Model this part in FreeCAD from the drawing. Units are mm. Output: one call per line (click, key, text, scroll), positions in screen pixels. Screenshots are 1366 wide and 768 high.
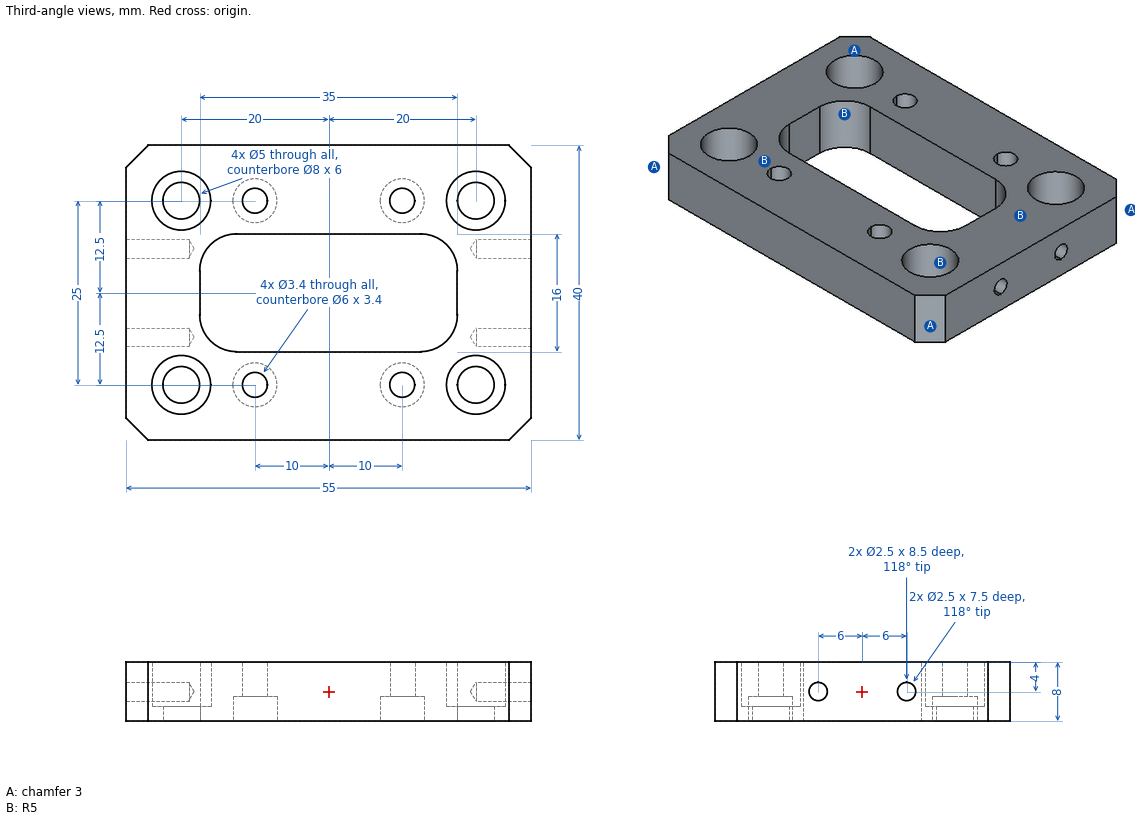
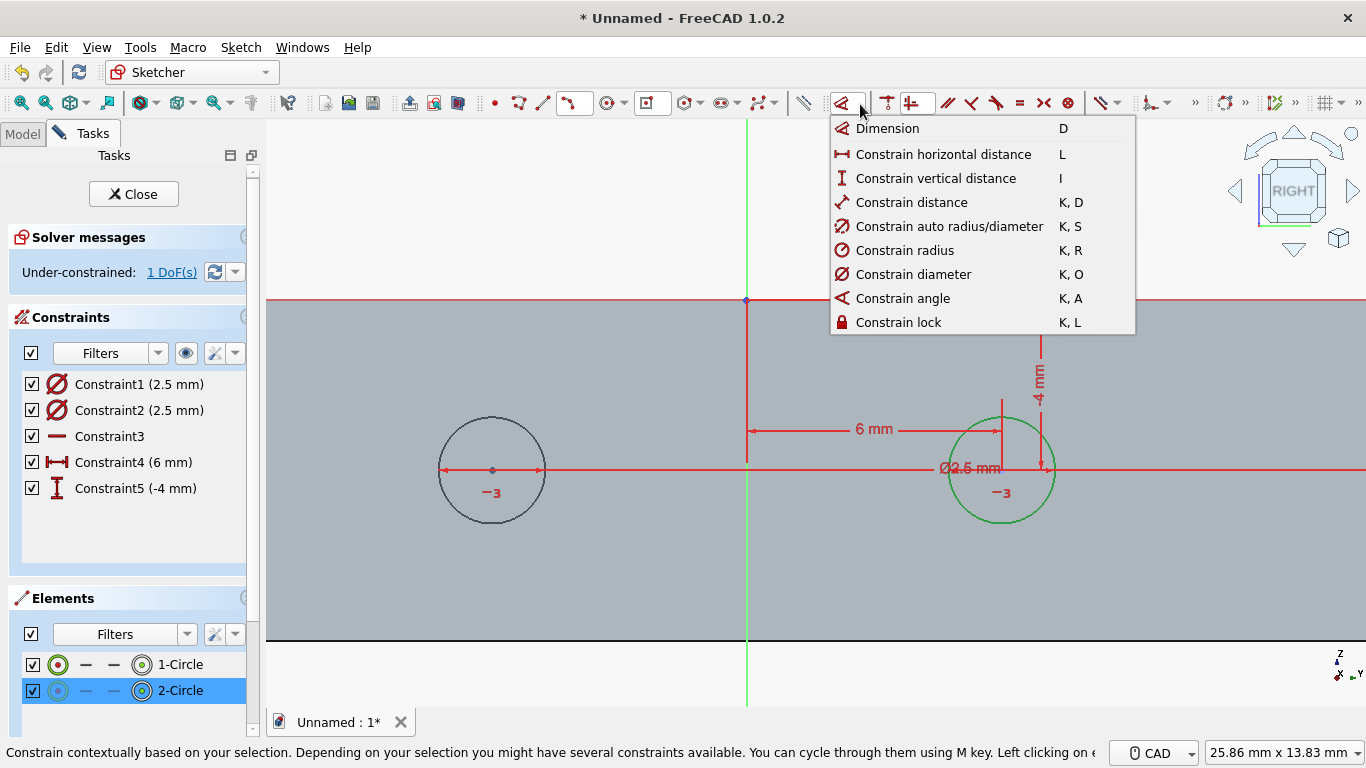
click(983, 154)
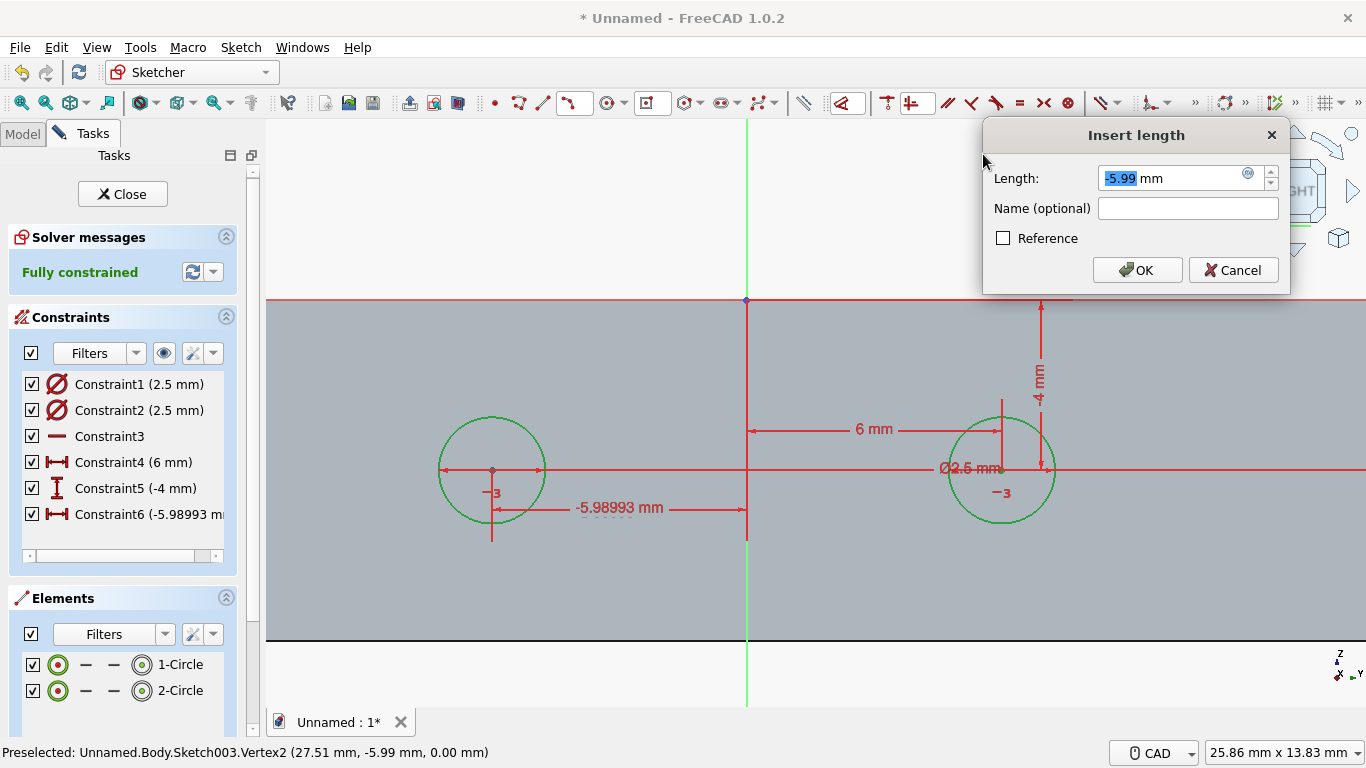
text(-6)
key(Return)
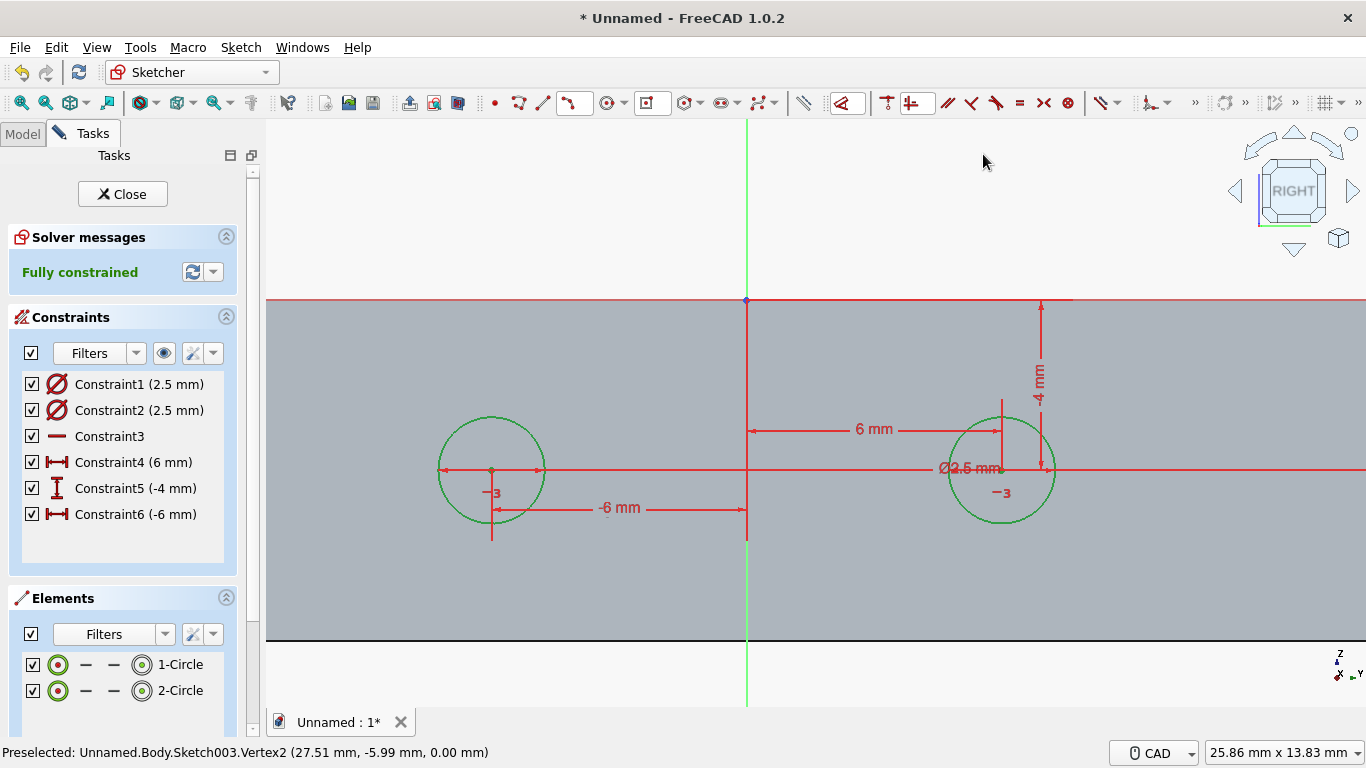
click(123, 194)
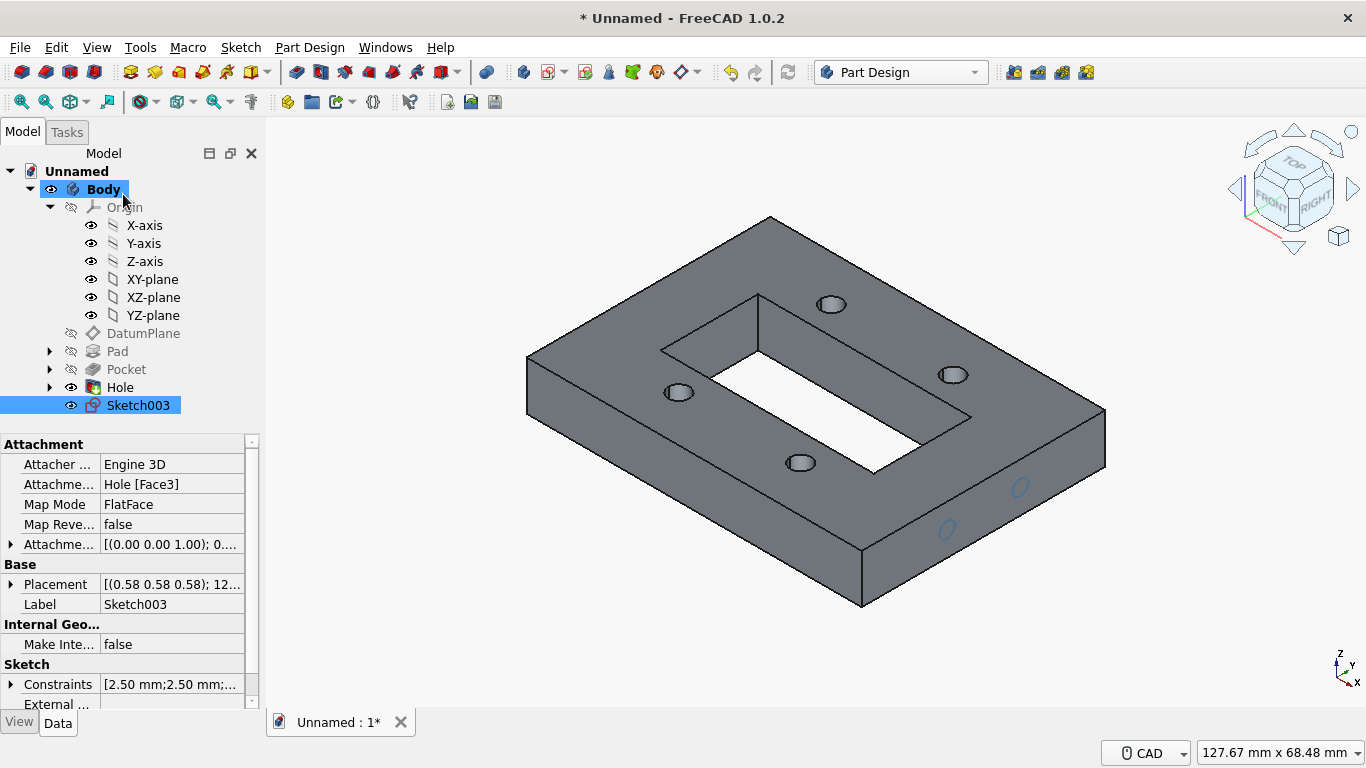
click(322, 72)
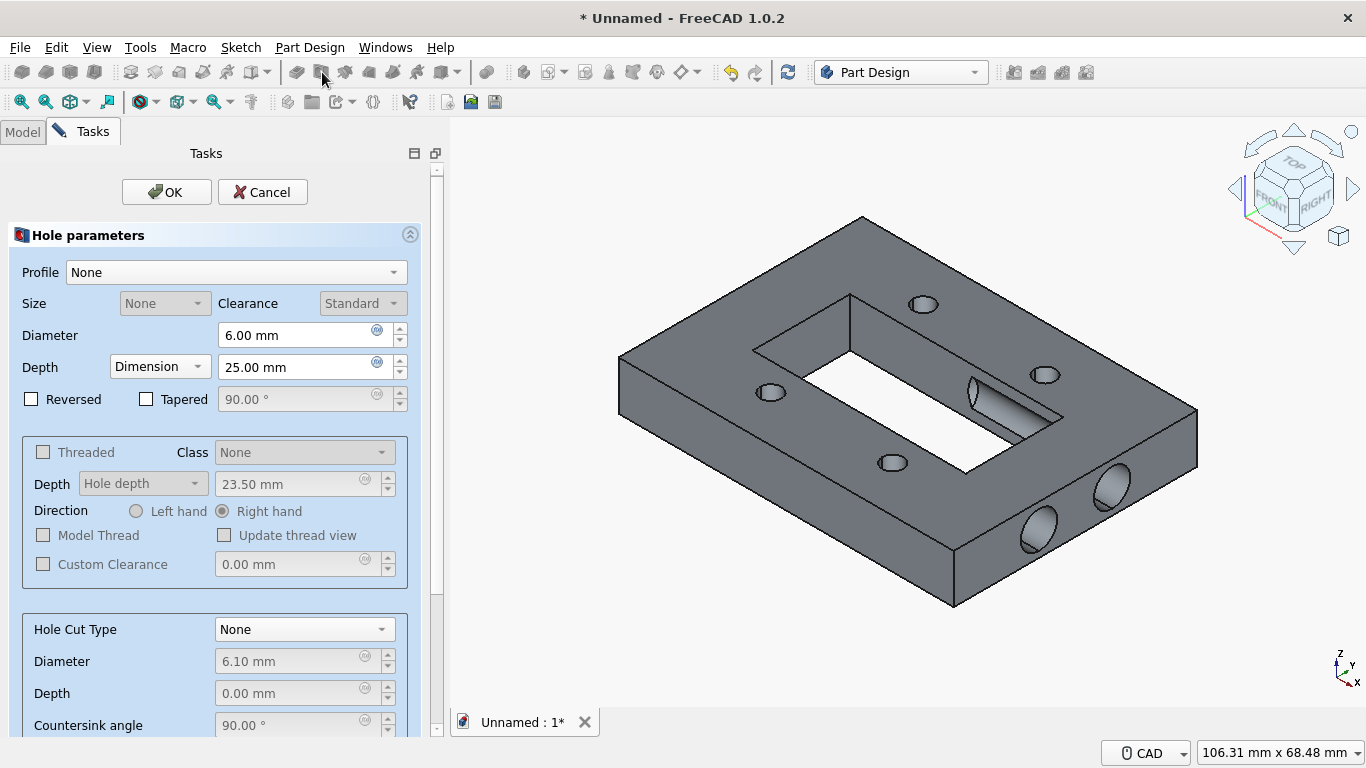
triple_click(305, 335)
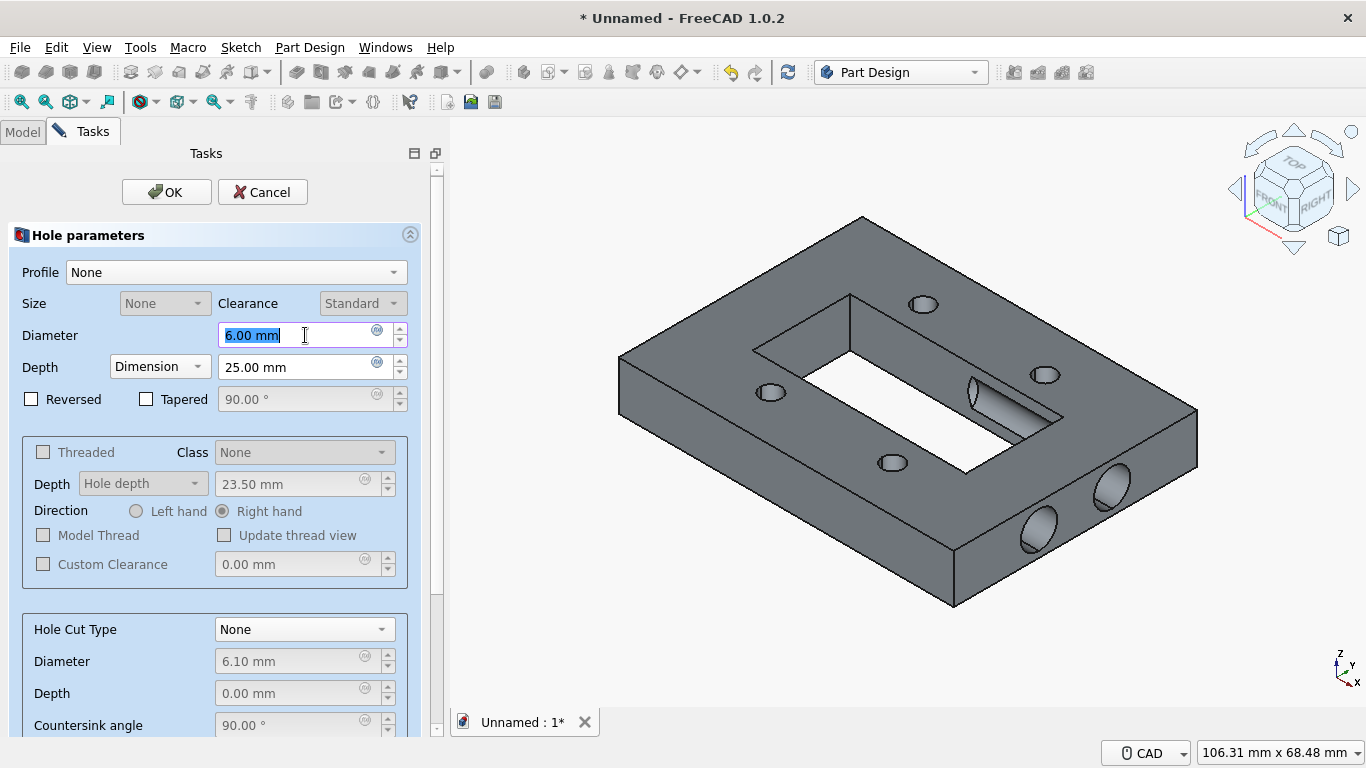
text(2.5)
key(Tab)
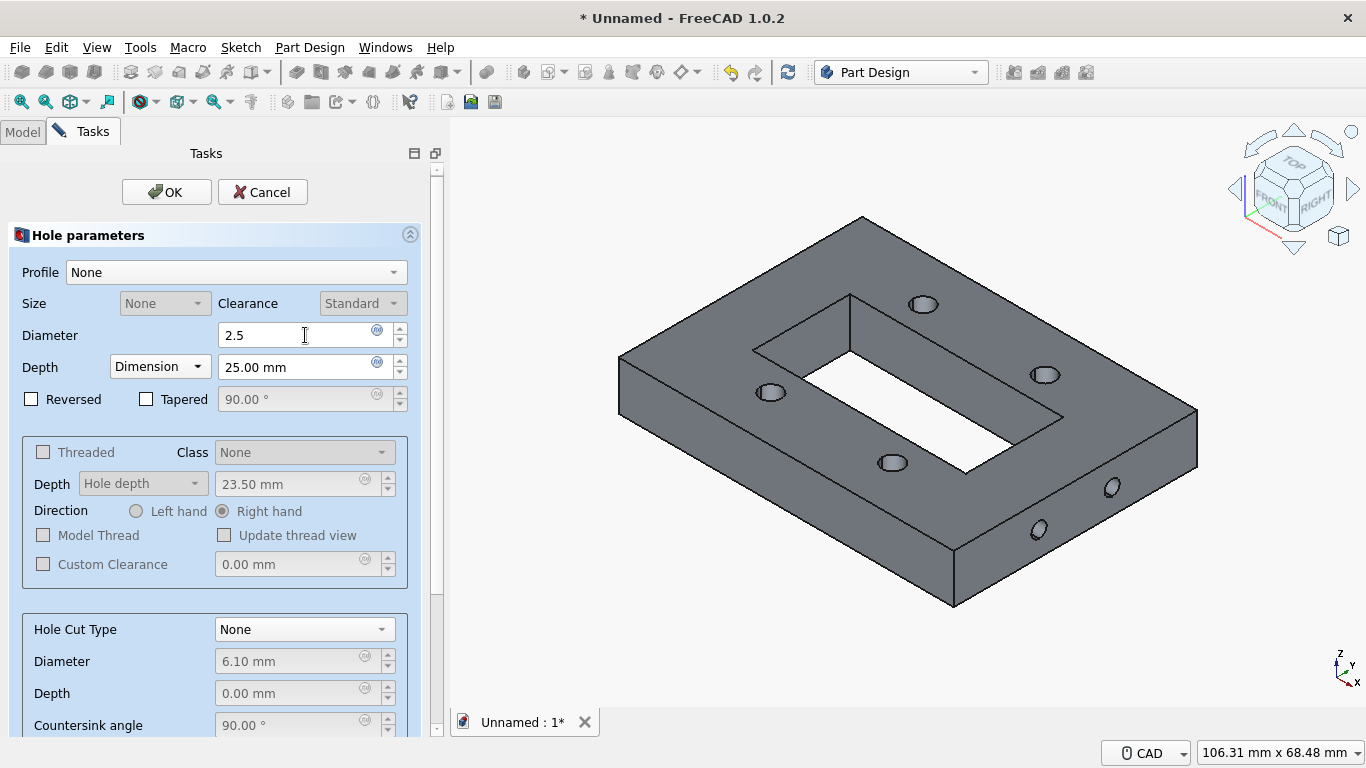
triple_click(305, 367)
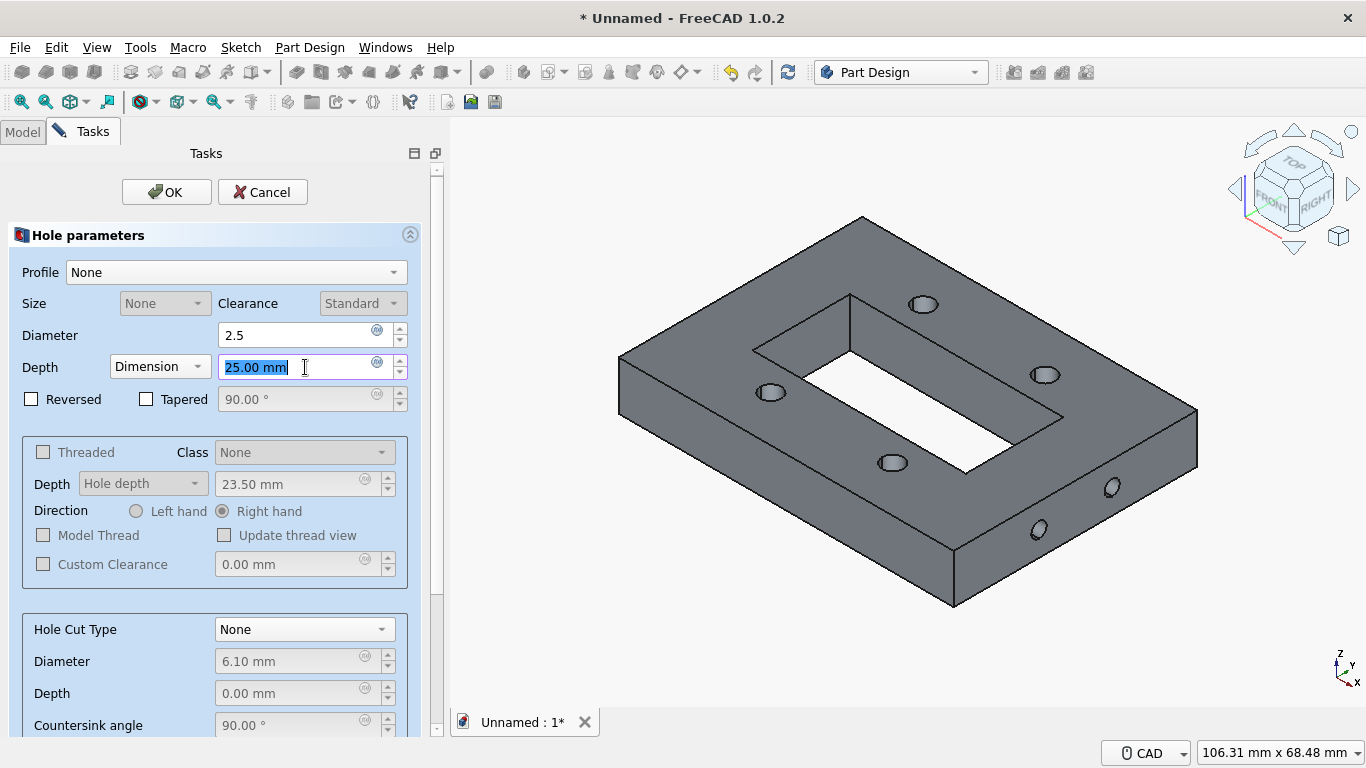
text(7.5)
key(Tab)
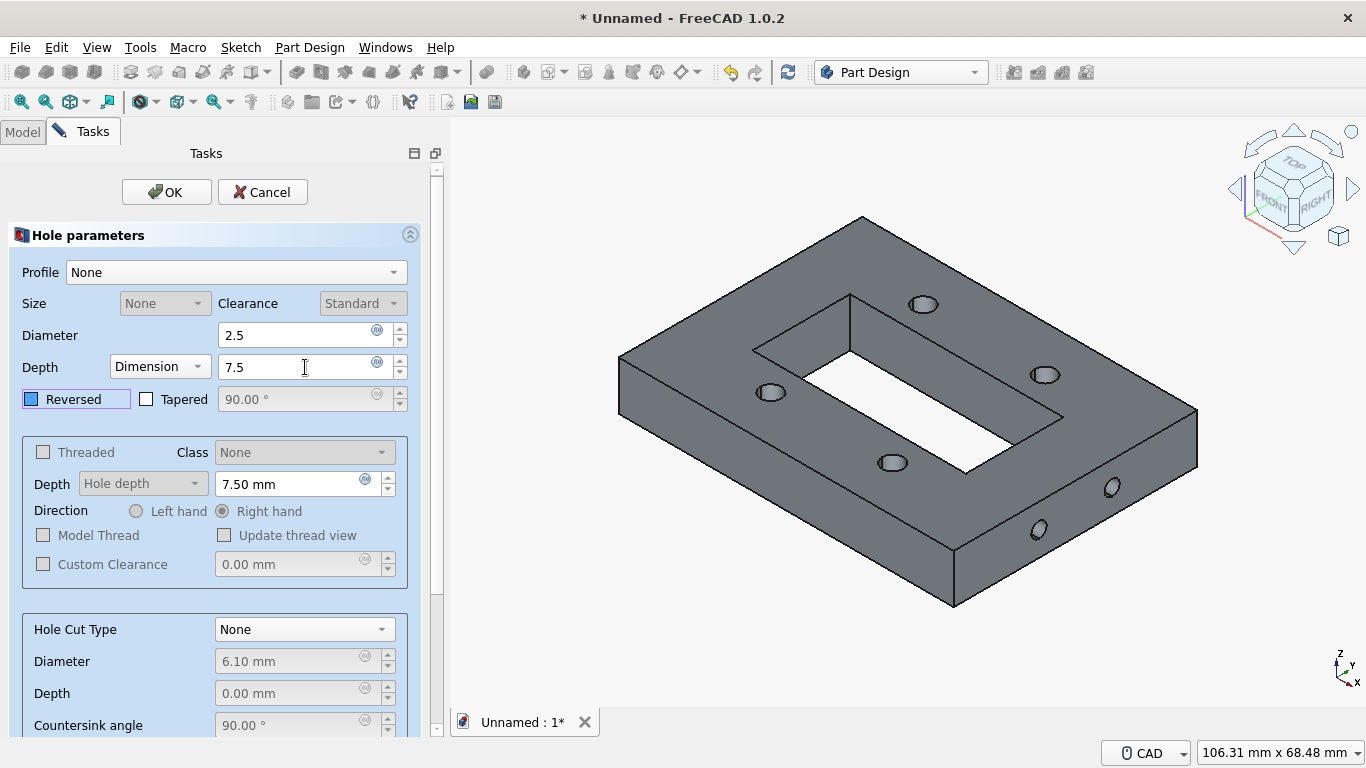
click(167, 192)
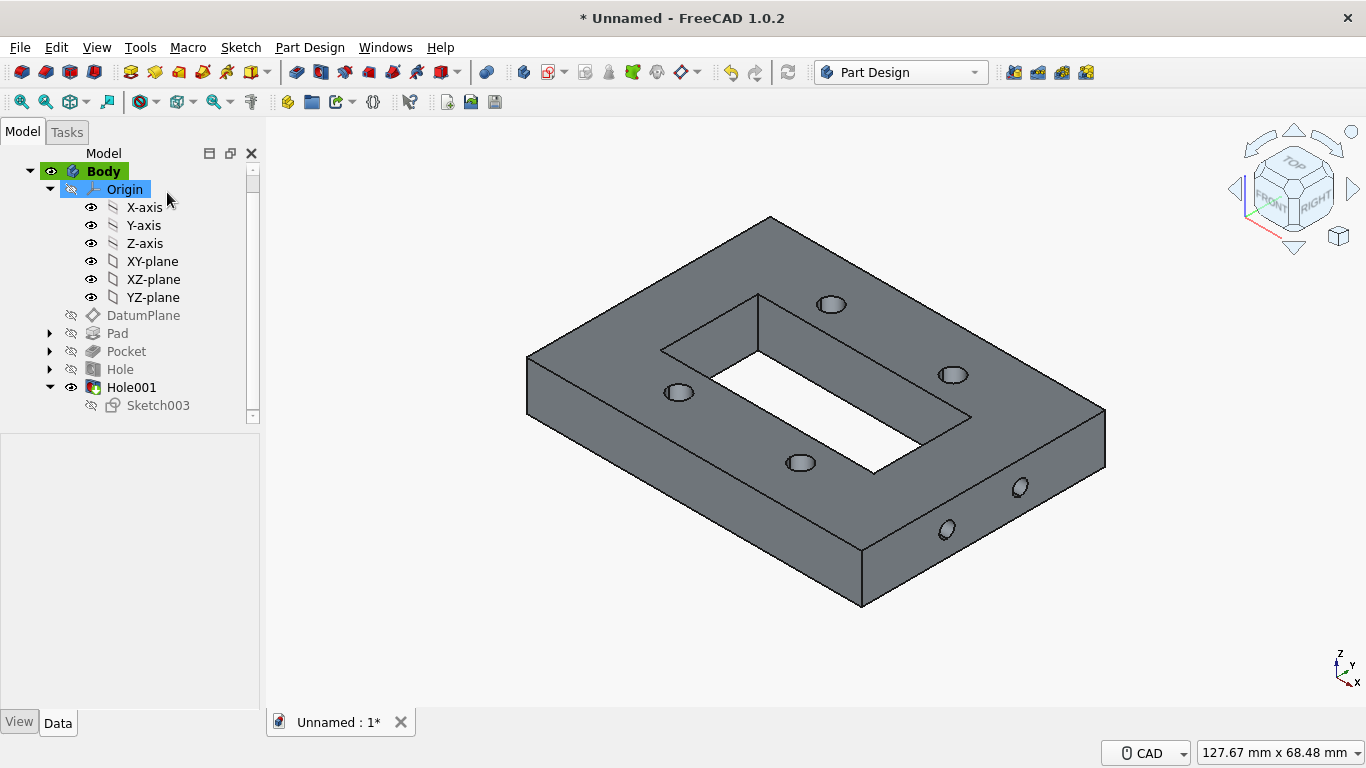
click(1029, 426)